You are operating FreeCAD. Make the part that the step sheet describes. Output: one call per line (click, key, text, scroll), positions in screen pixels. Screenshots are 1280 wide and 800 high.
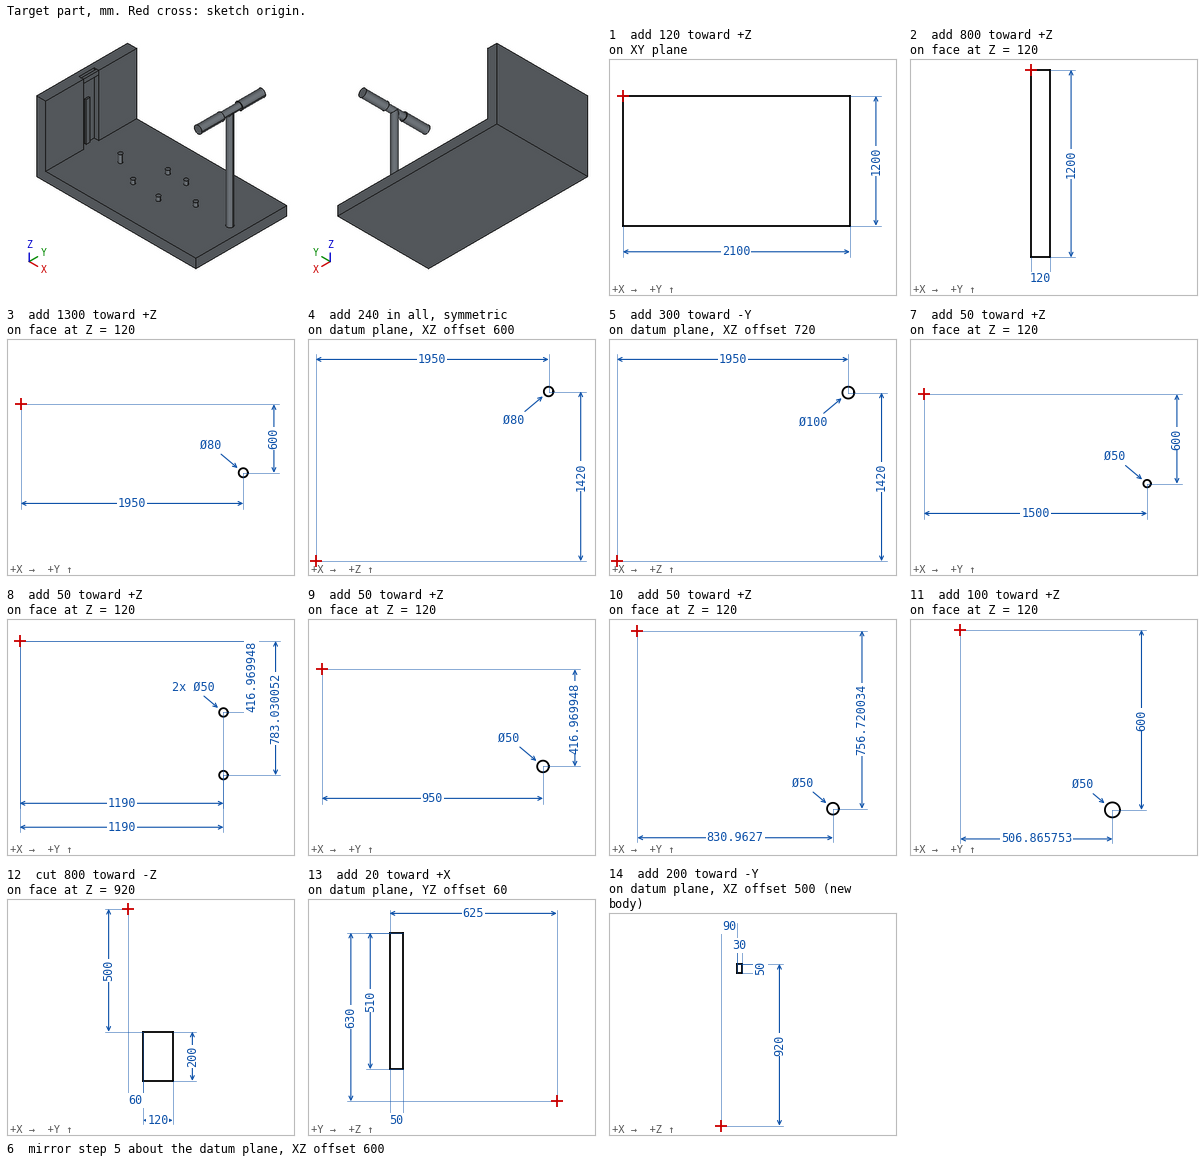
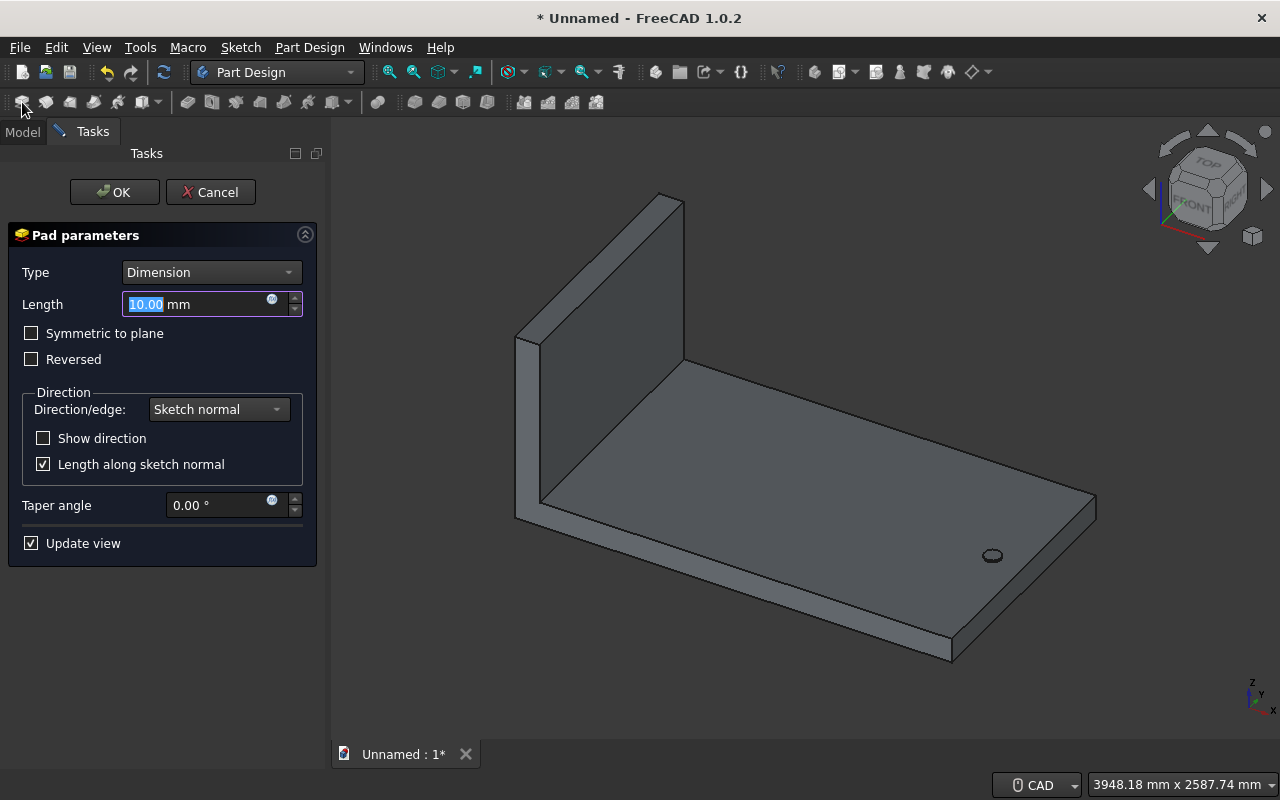
text(1300)
key(Tab)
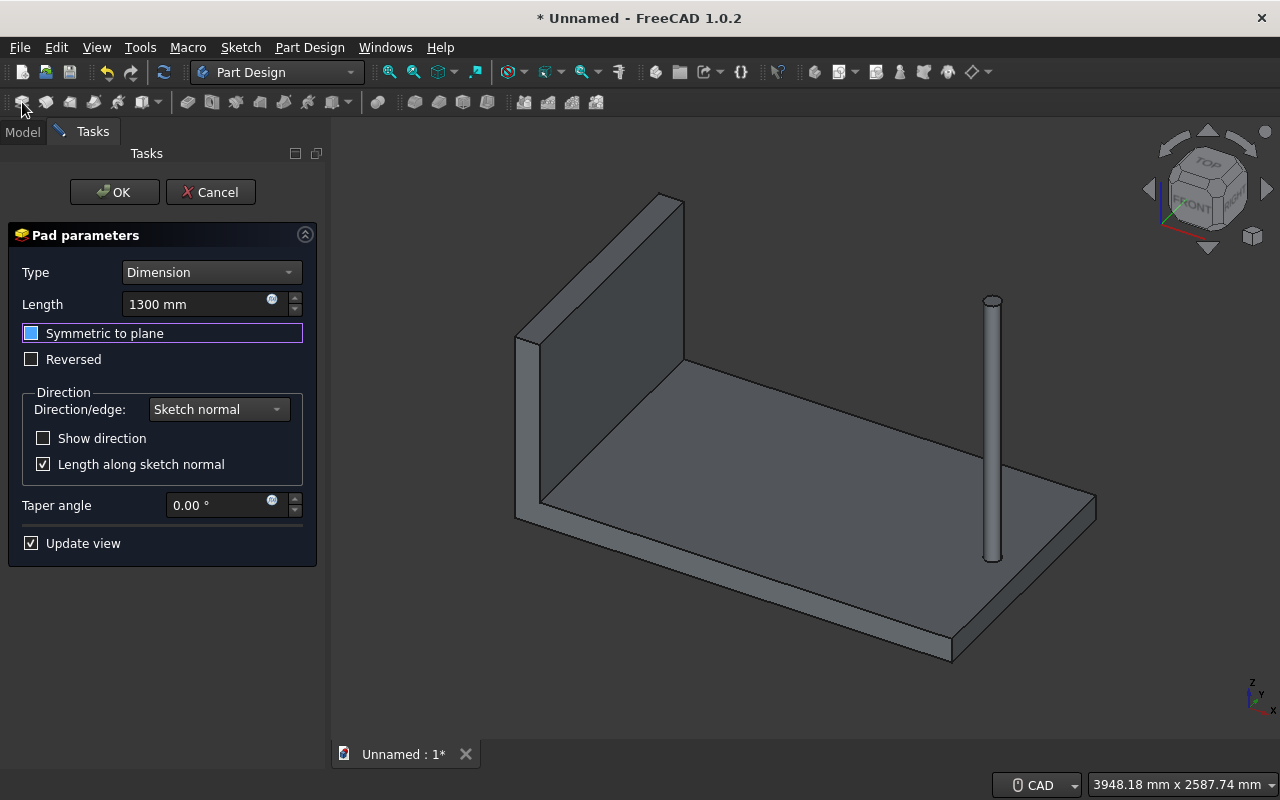
click(115, 192)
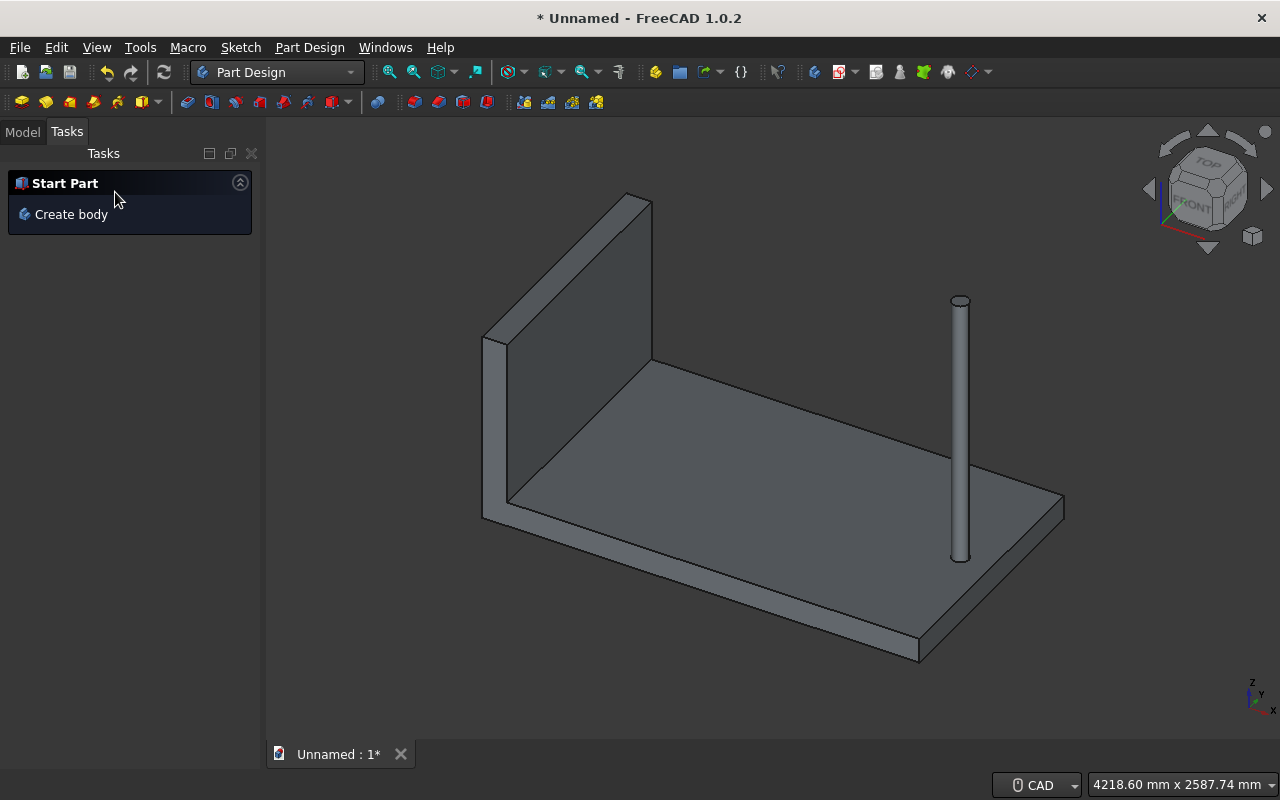
click(390, 72)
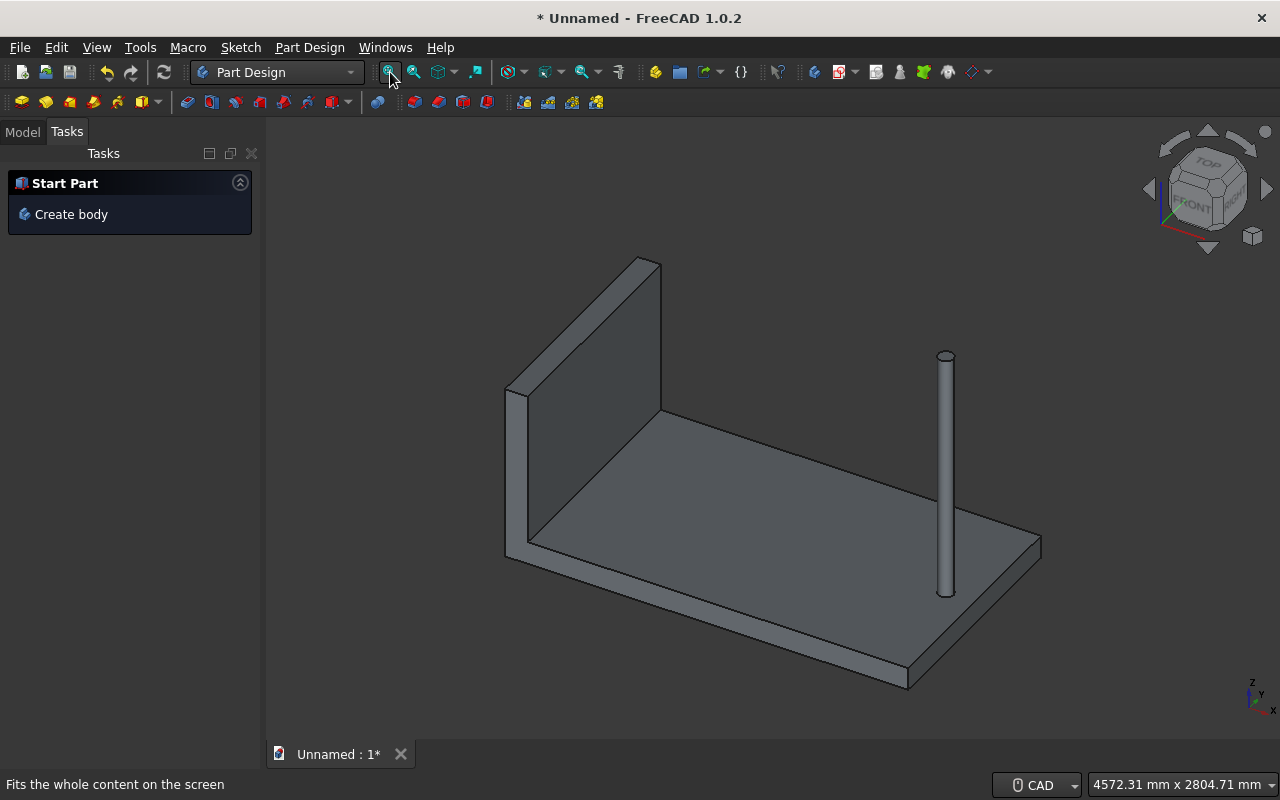
click(23, 131)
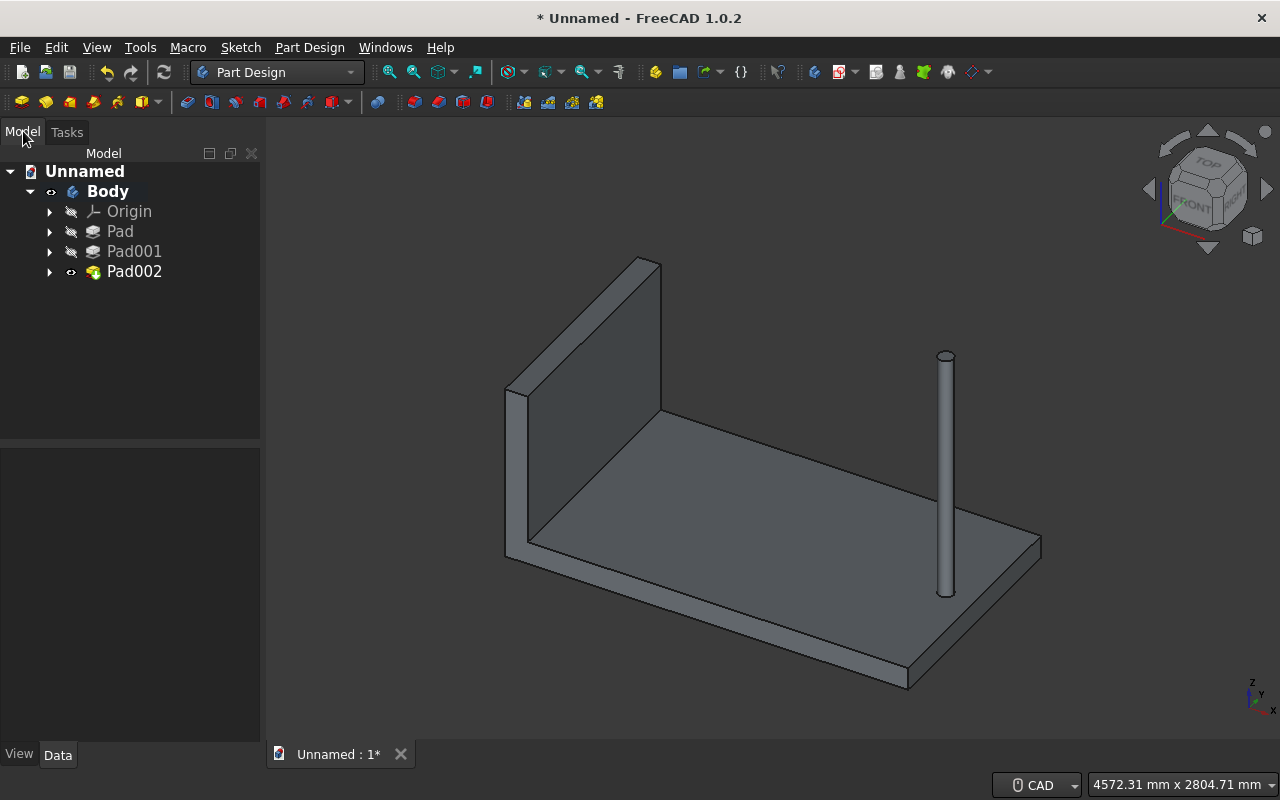
click(50, 212)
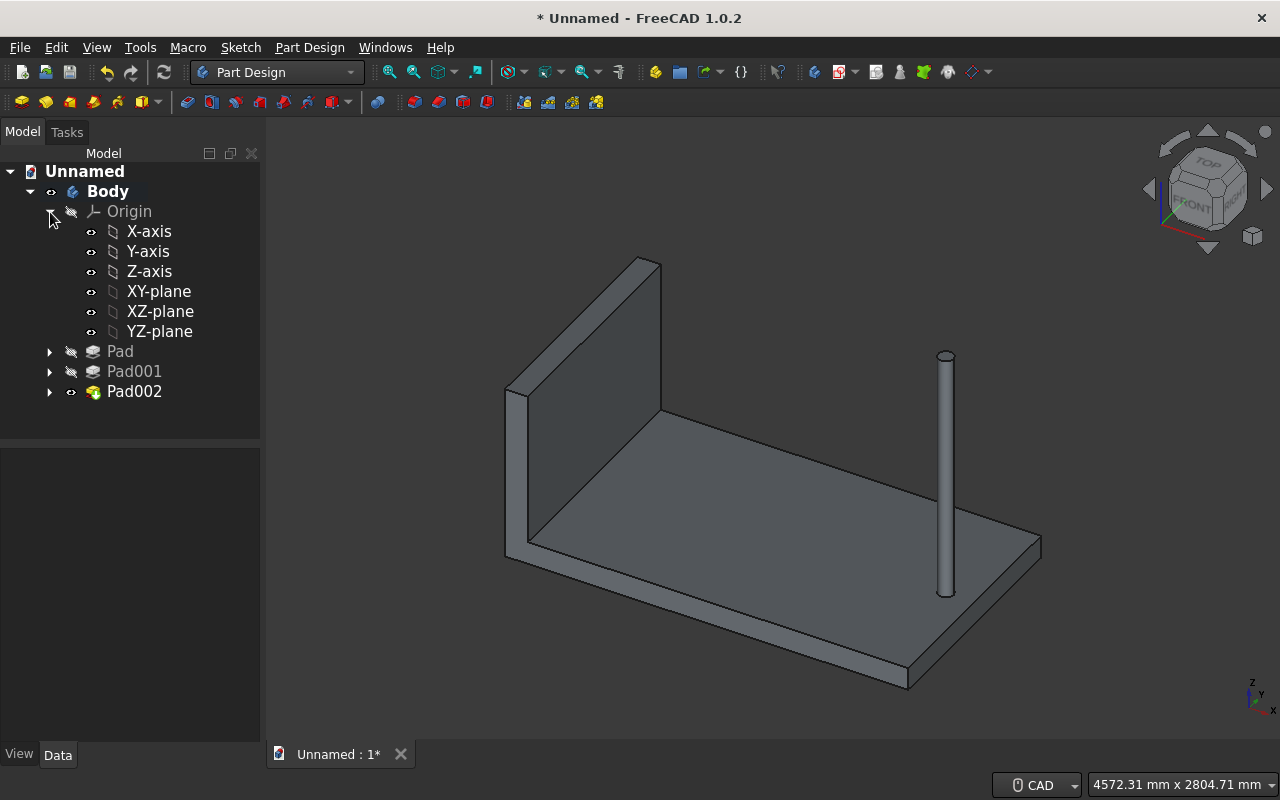
click(136, 312)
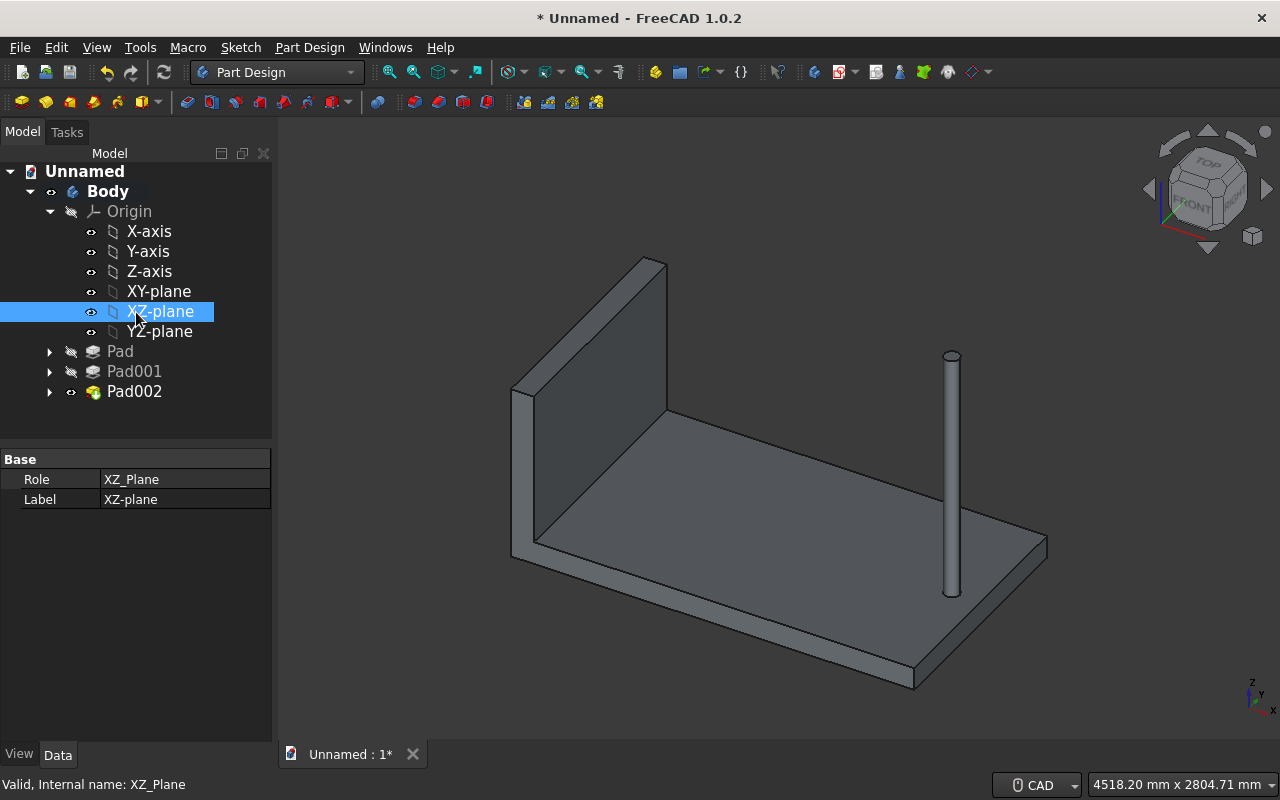
click(972, 72)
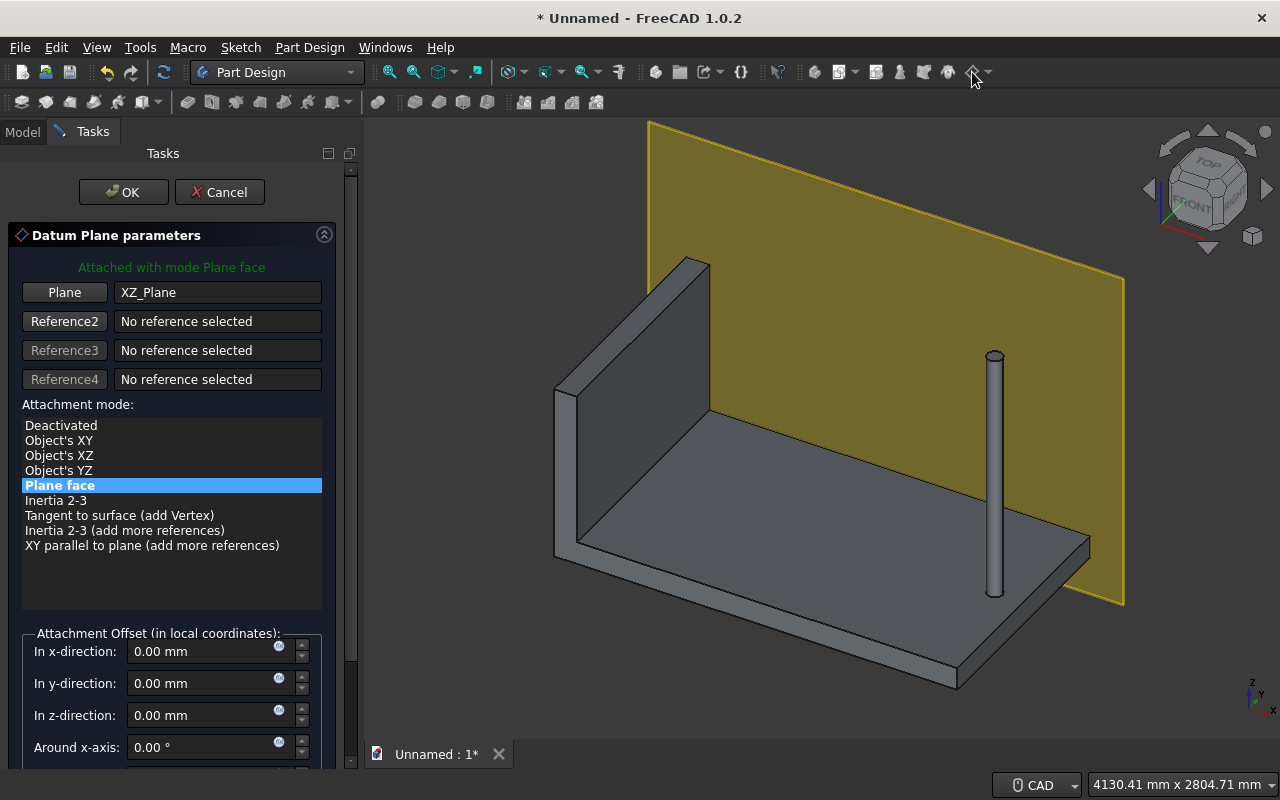
triple_click(210, 715)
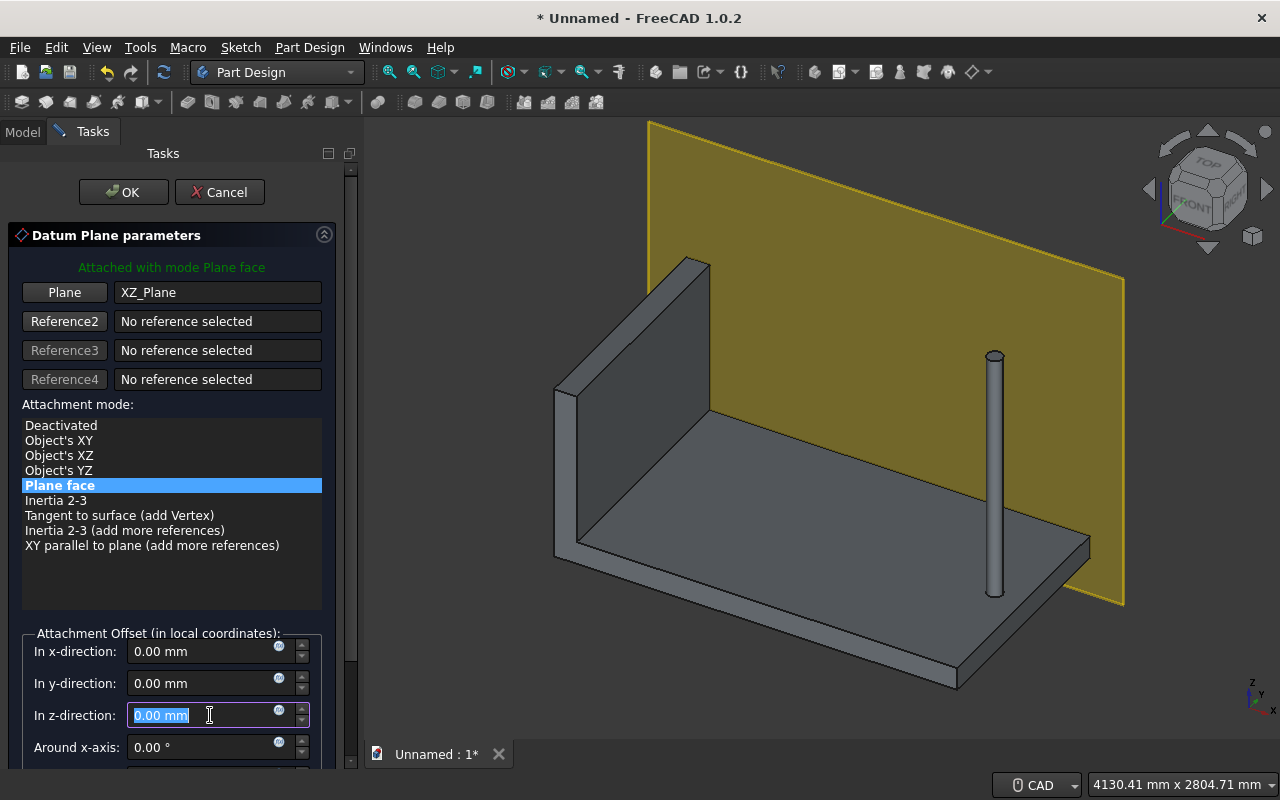
text(600)
key(Tab)